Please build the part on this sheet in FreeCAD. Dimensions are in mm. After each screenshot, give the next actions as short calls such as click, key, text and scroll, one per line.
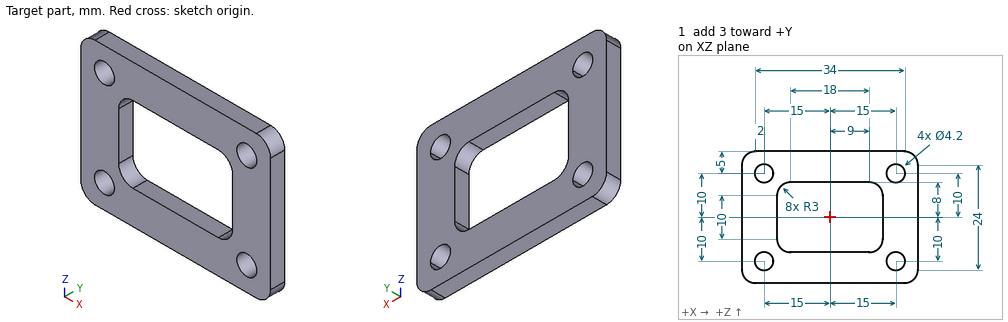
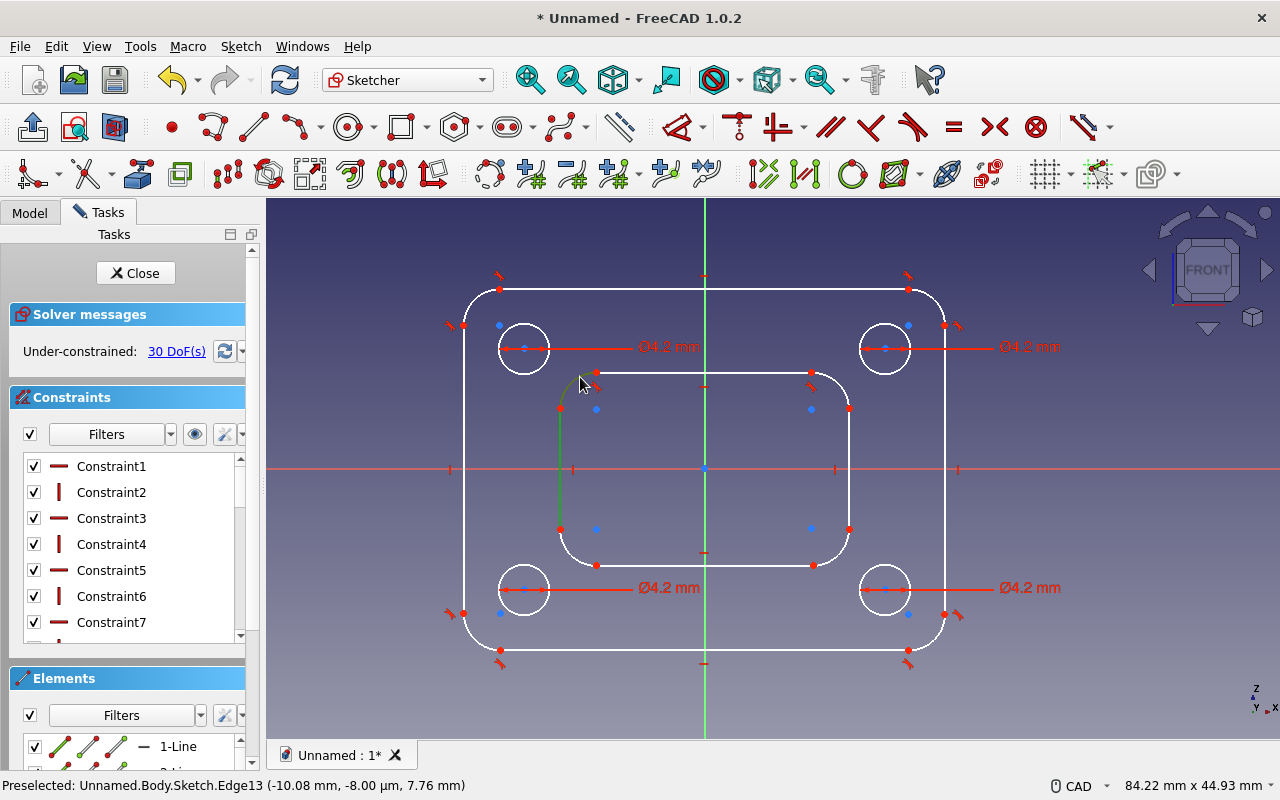
key(t)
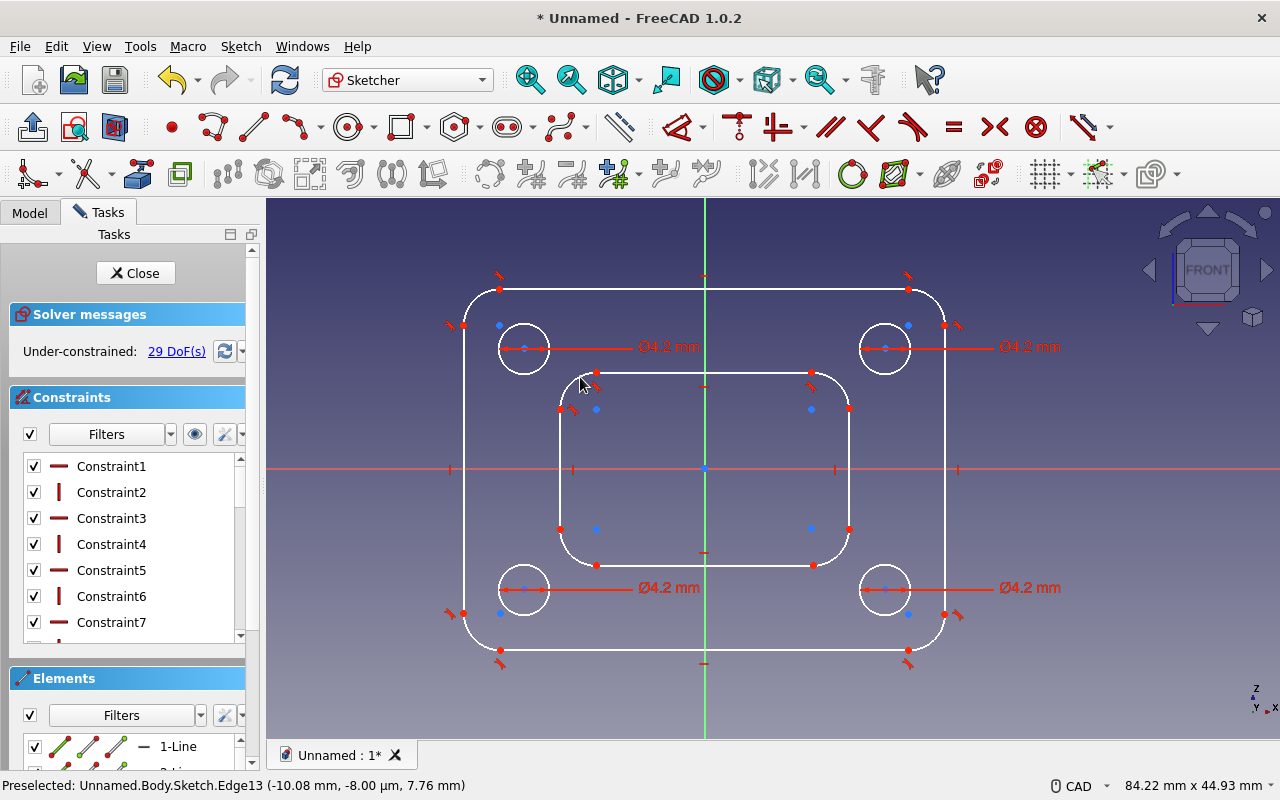
click(560, 445)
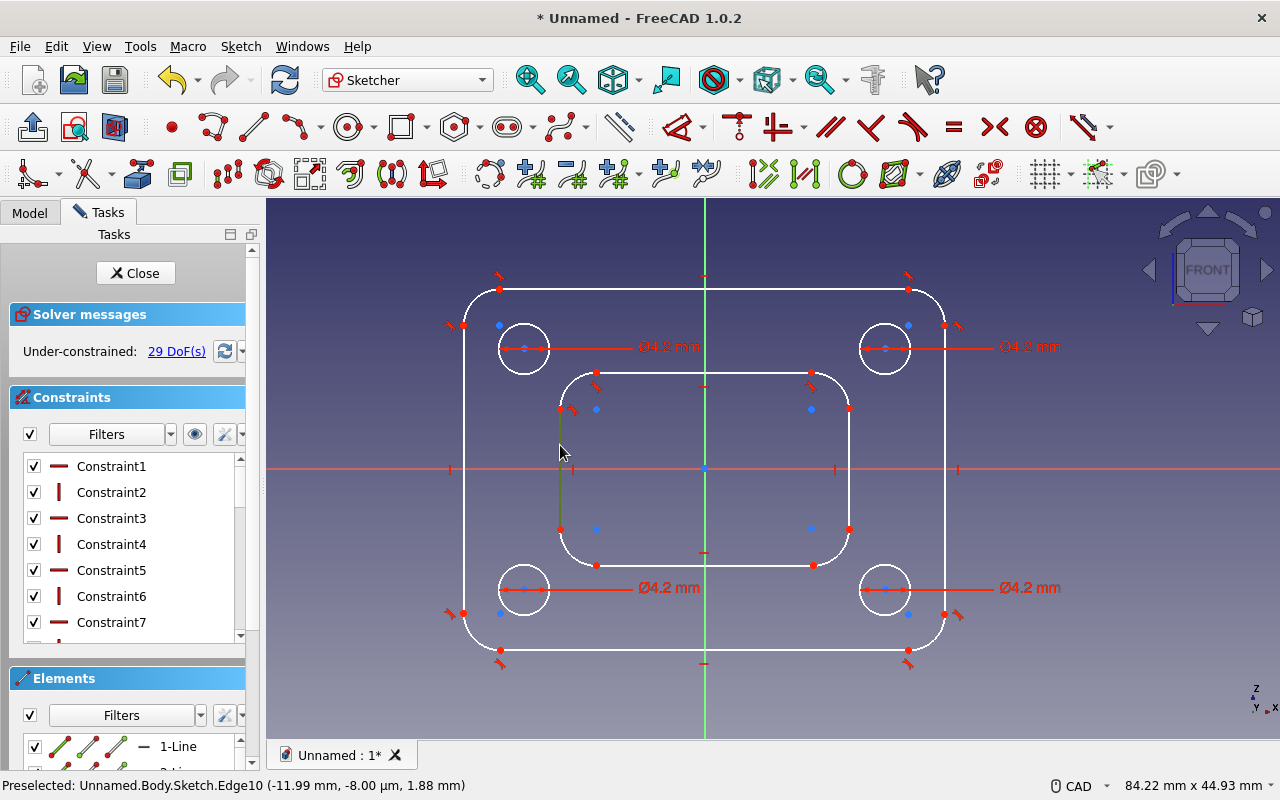
click(564, 546)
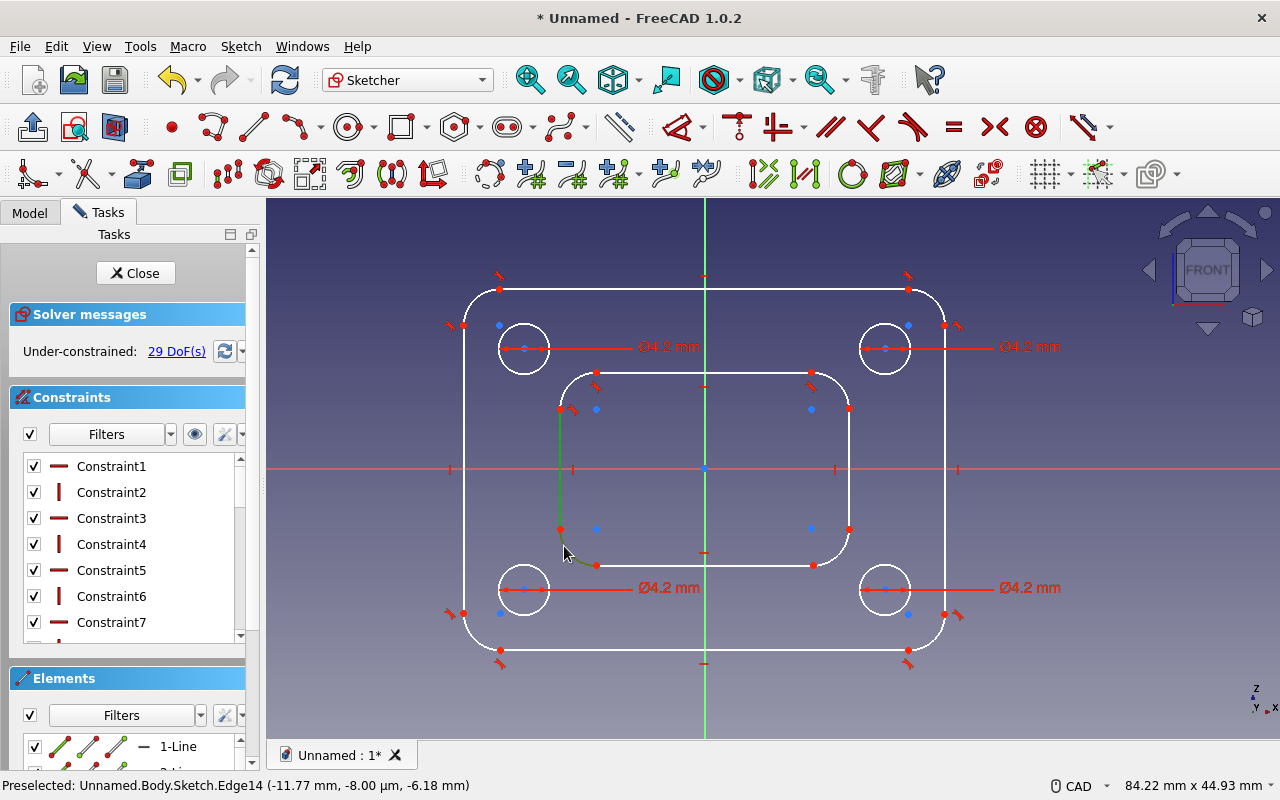
click(913, 128)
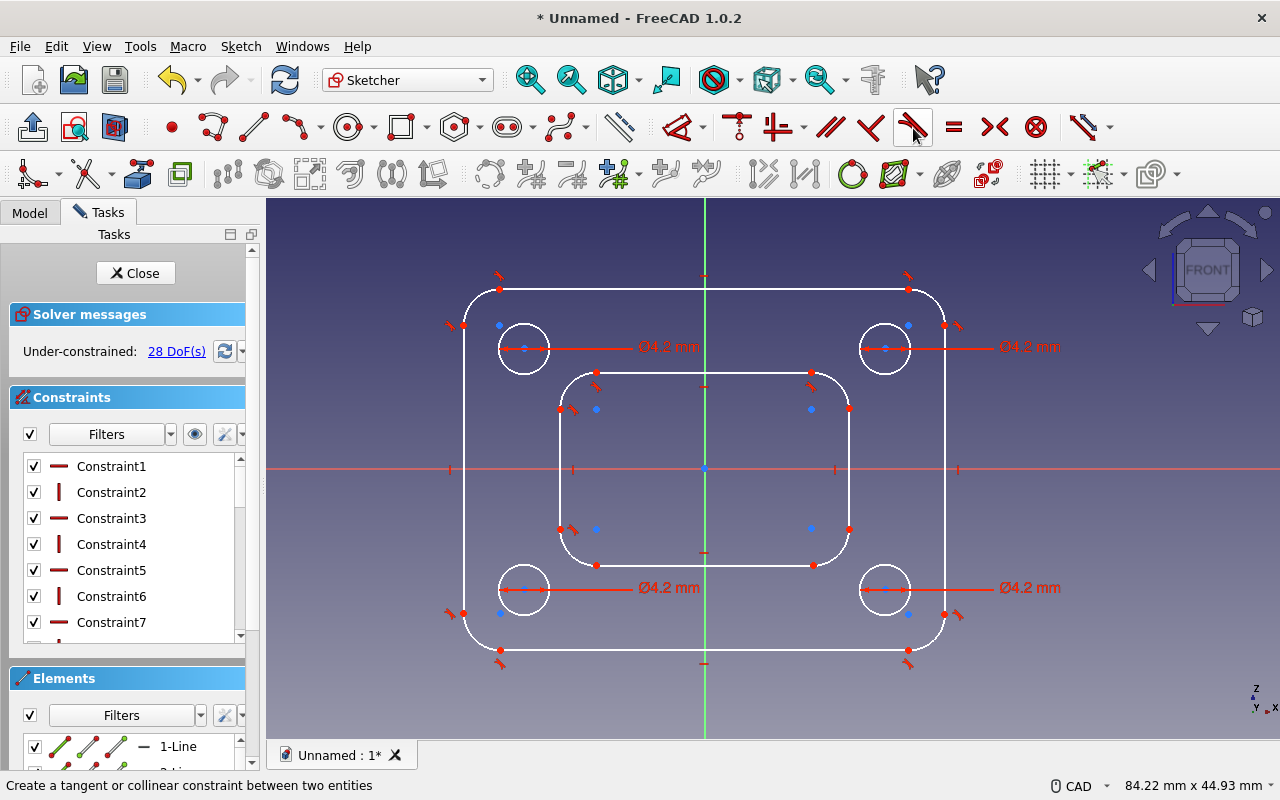
click(661, 566)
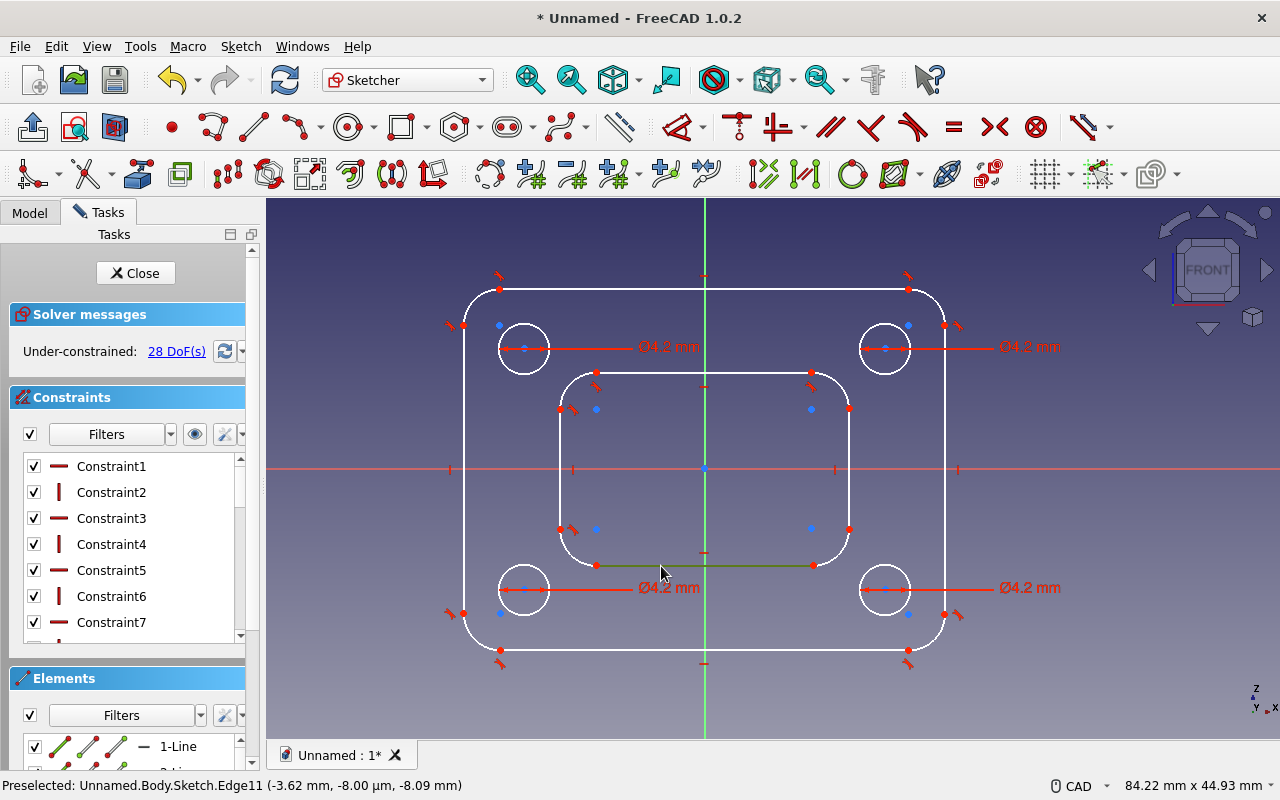
click(564, 546)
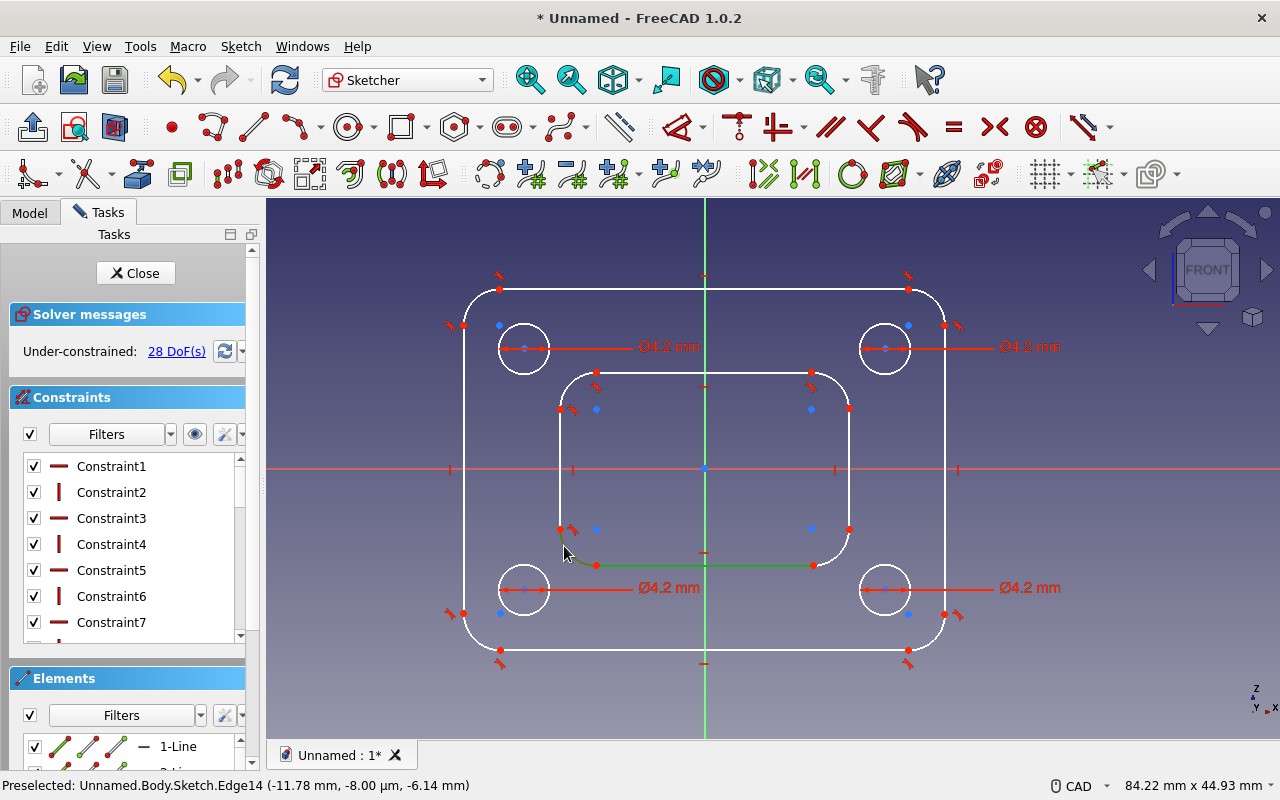
click(913, 128)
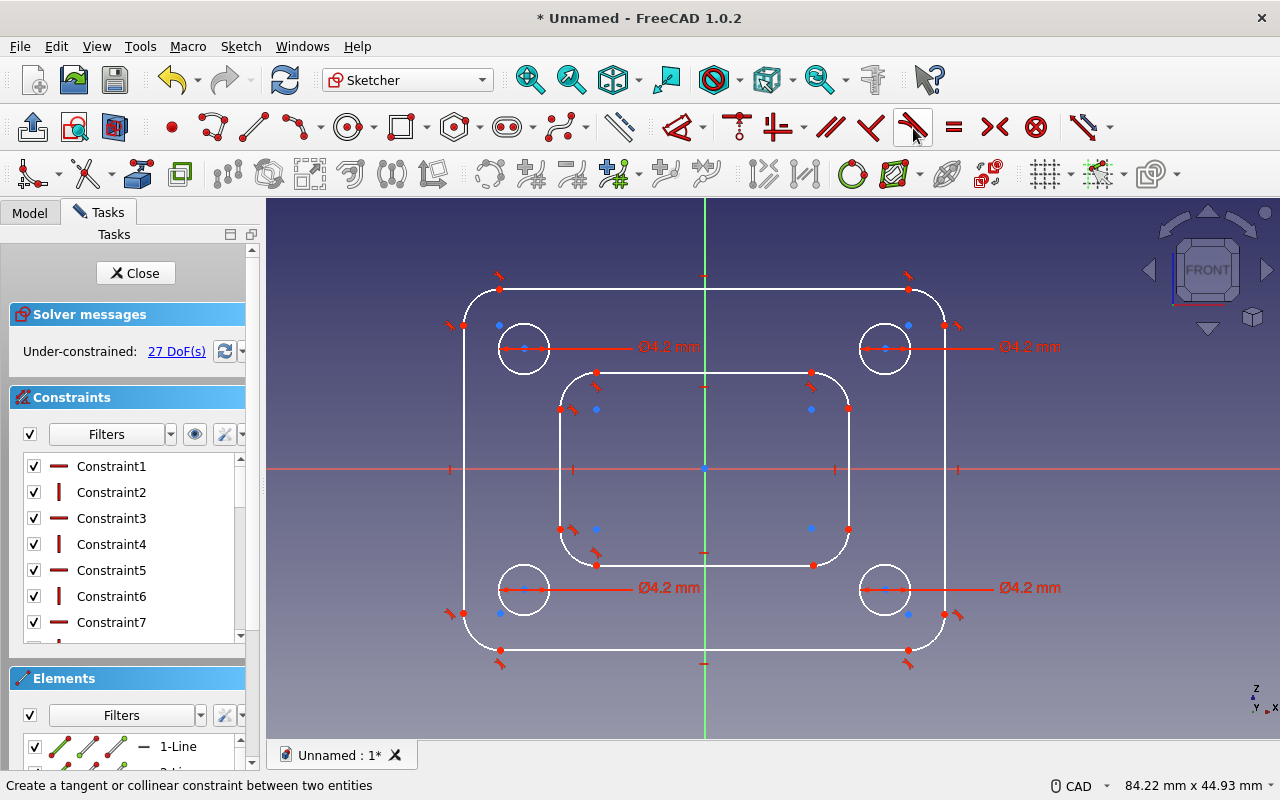
click(662, 566)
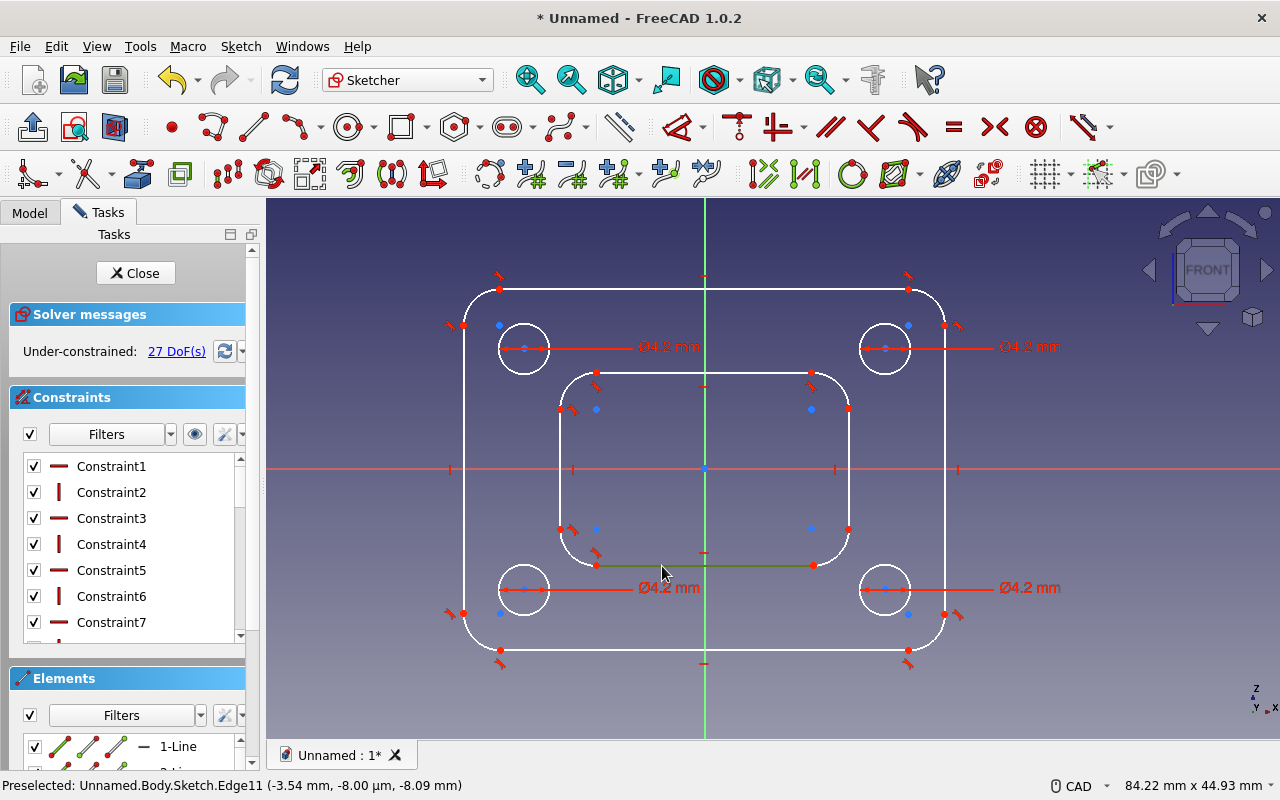
click(829, 562)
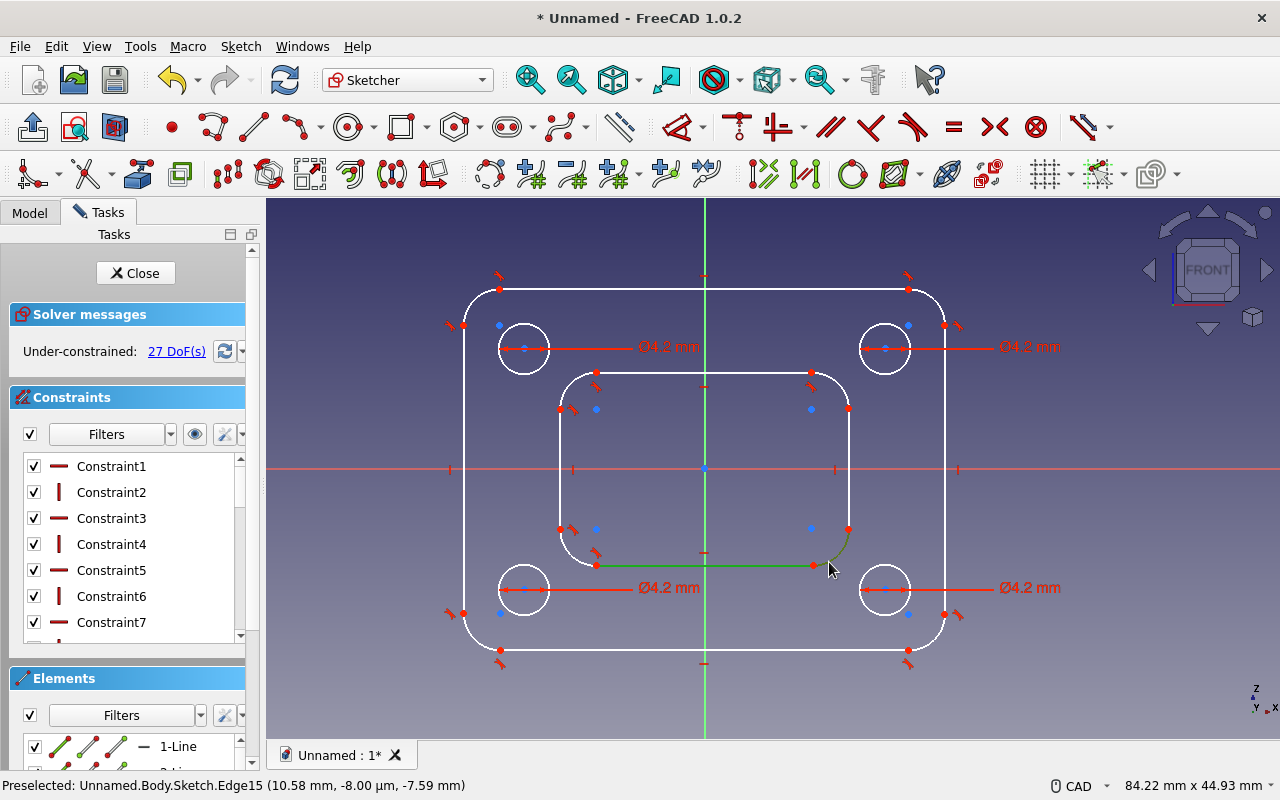
key(t)